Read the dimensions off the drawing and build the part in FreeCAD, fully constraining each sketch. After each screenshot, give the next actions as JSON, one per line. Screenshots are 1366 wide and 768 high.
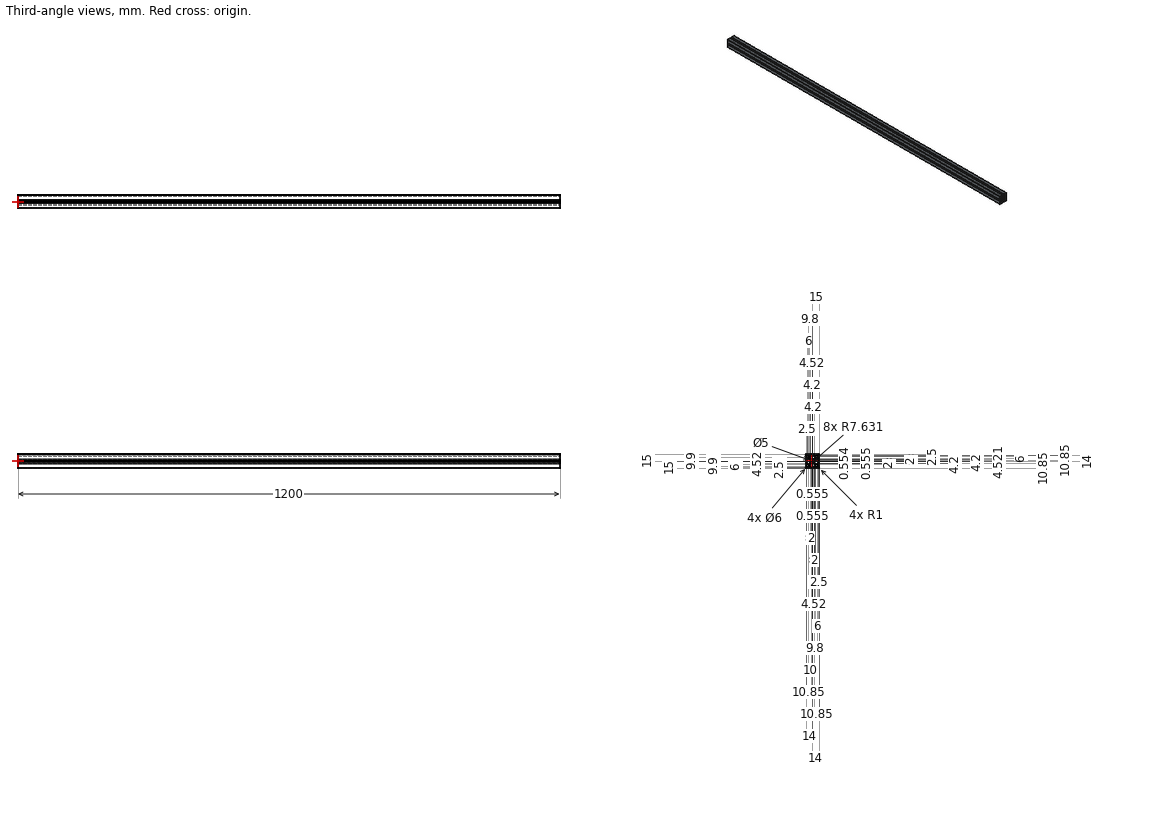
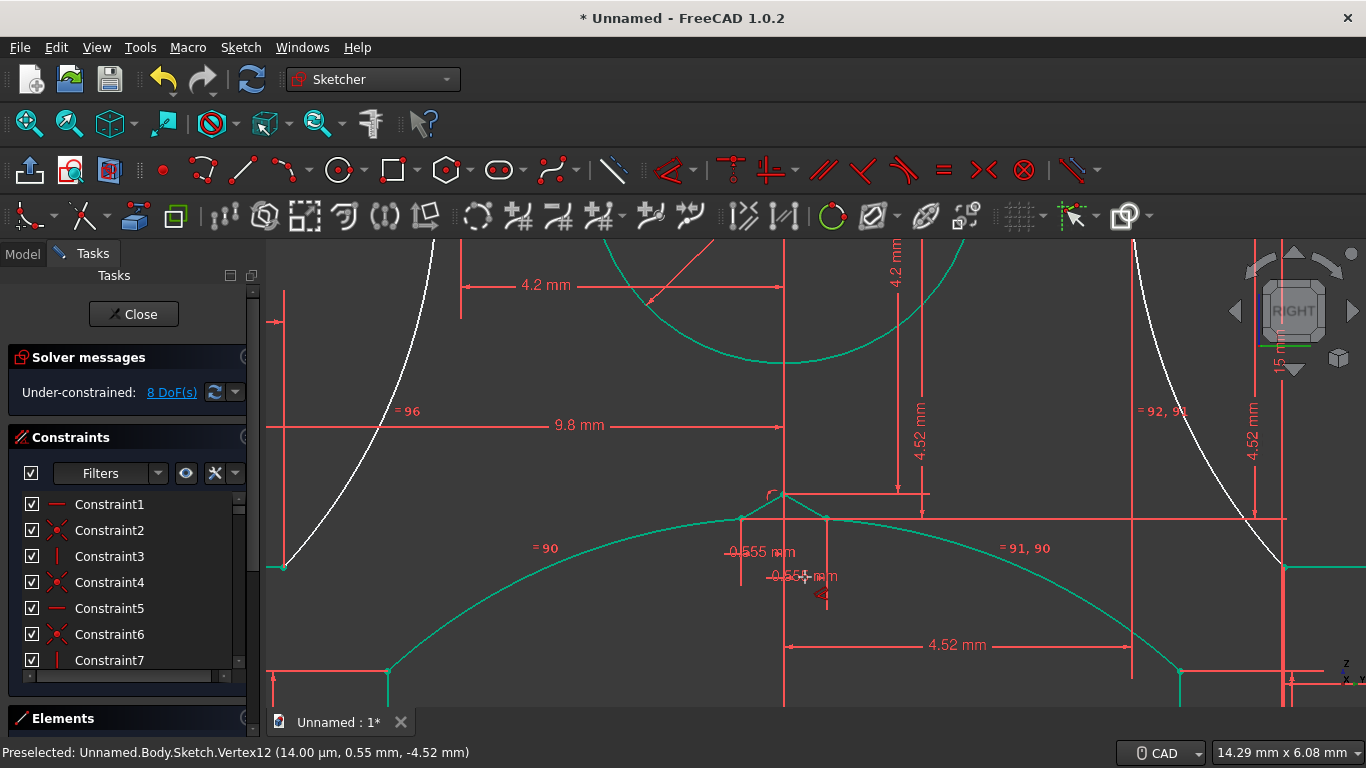
{"action": "scroll", "coordinate": [742, 520], "scroll_direction": "down", "scroll_amount": 10}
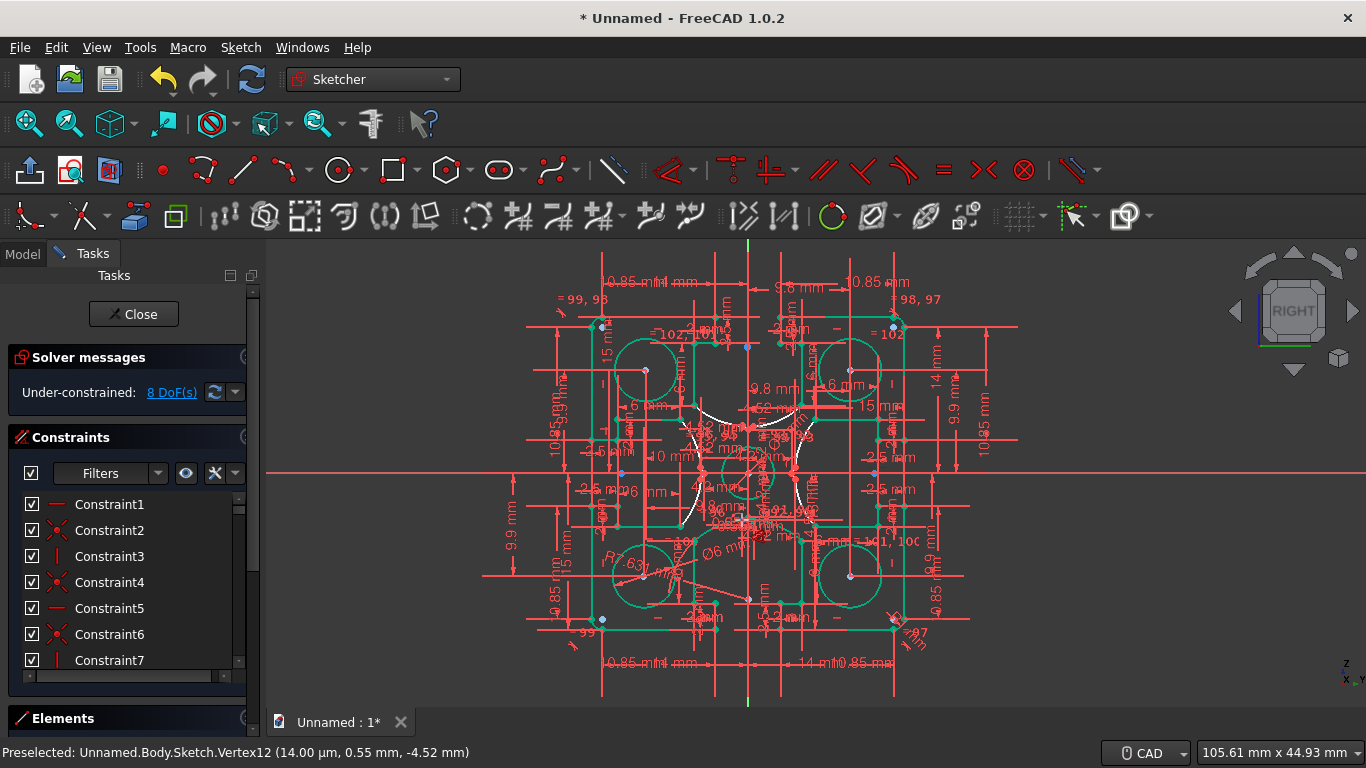
{"action": "scroll", "coordinate": [795, 479], "scroll_direction": "up", "scroll_amount": 10}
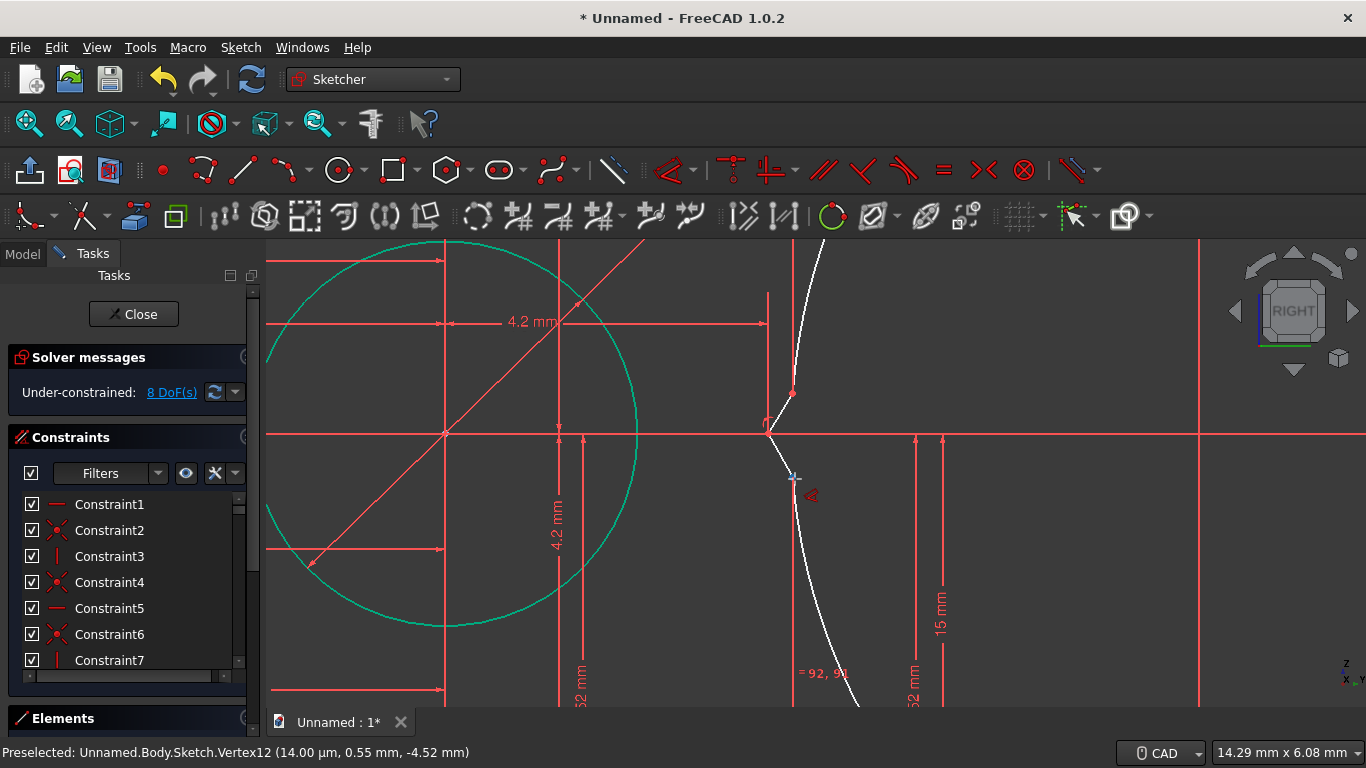
{"action": "left_click", "coordinate": [793, 477]}
{"action": "left_click", "coordinate": [827, 455]}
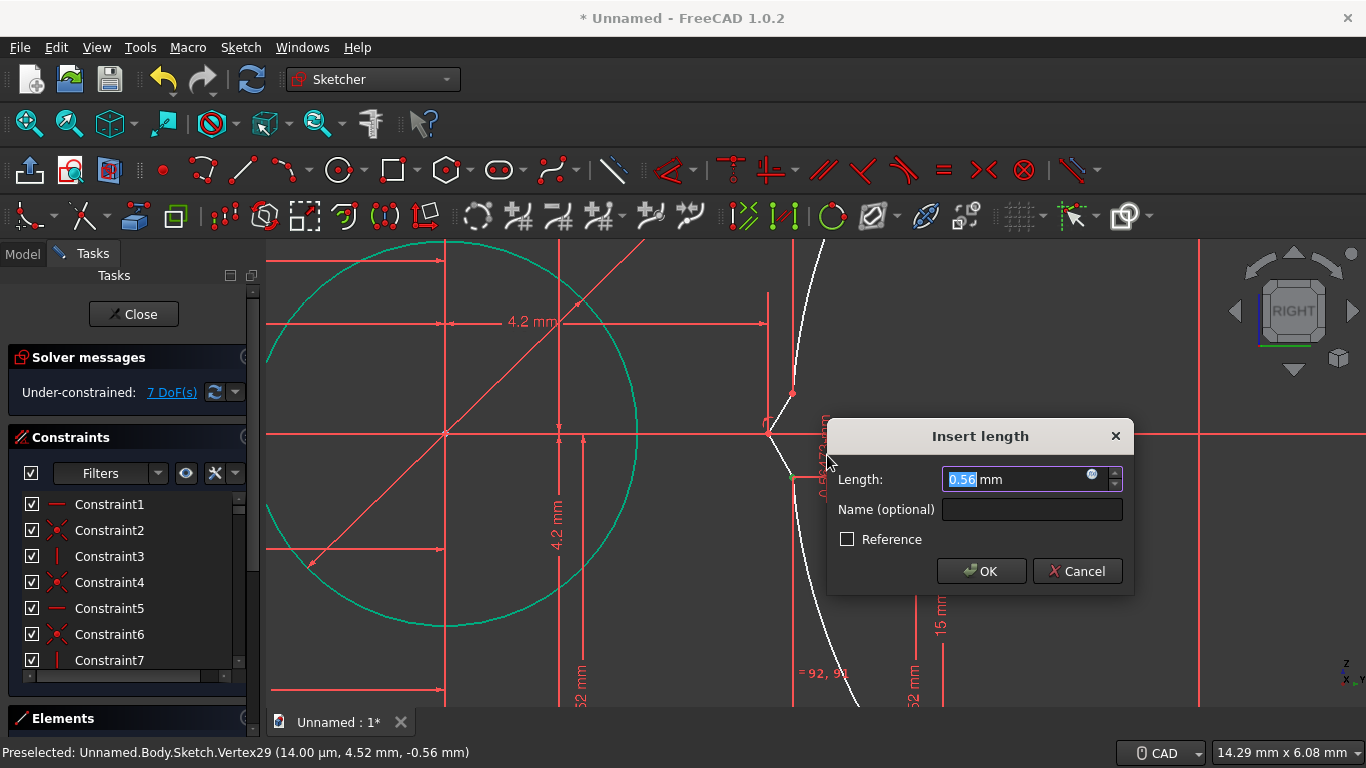
{"action": "type", "text": "0.554"}
{"action": "key", "text": "Return"}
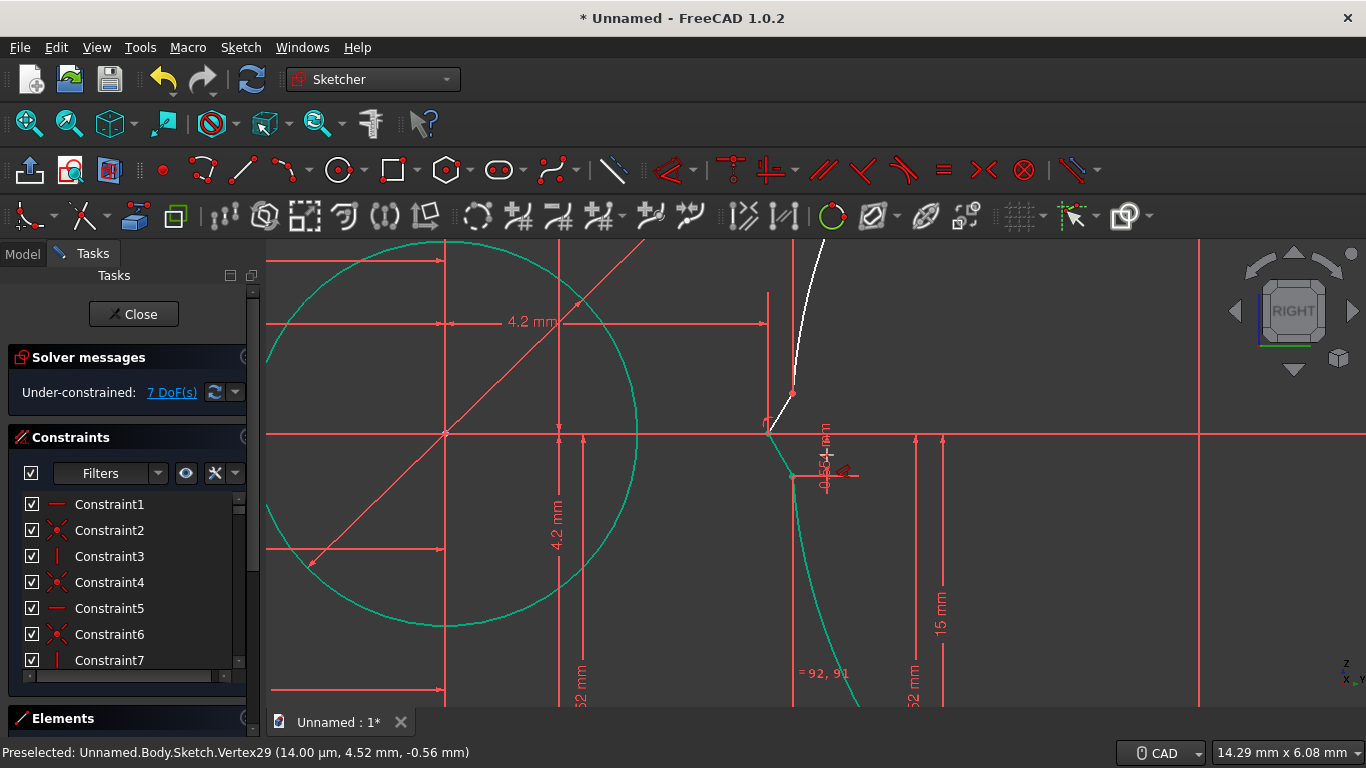
{"action": "left_click", "coordinate": [793, 393]}
{"action": "left_click", "coordinate": [827, 413]}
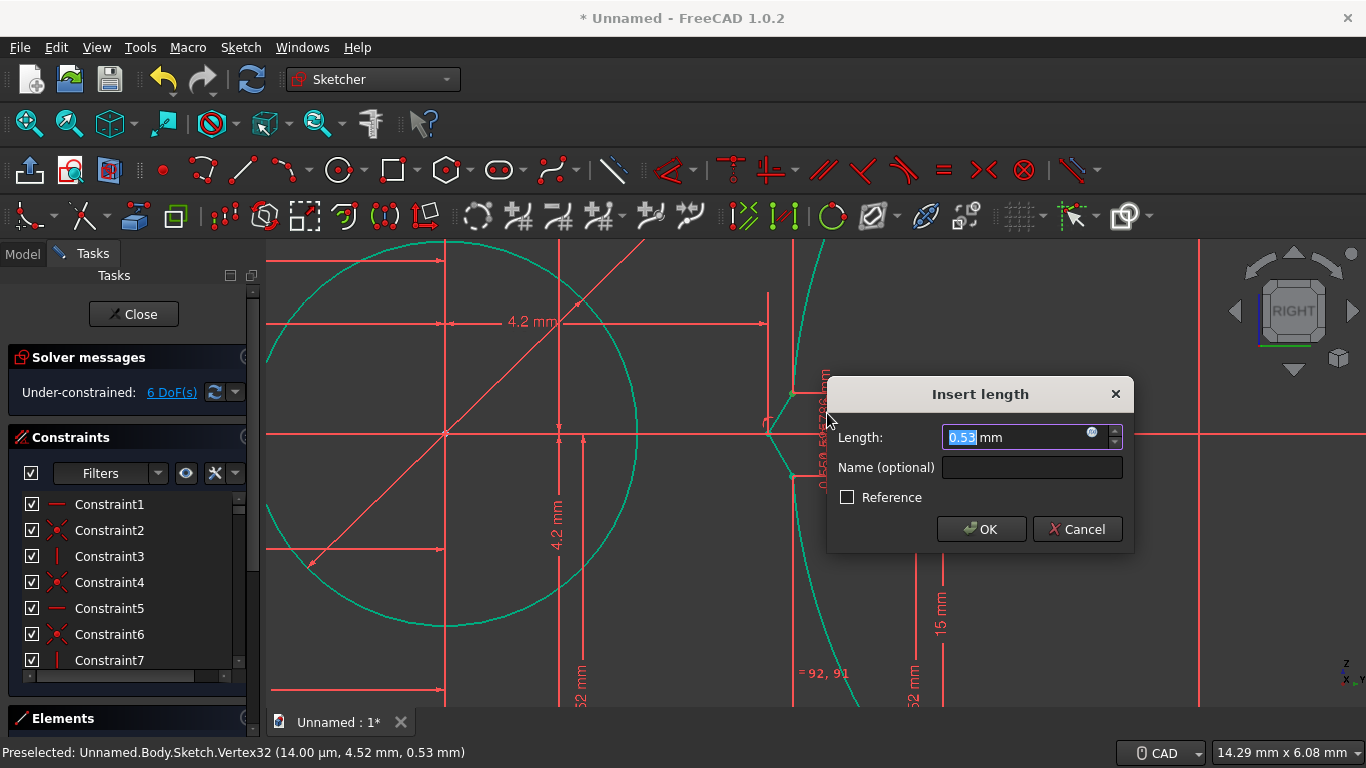
{"action": "type", "text": "0.555"}
{"action": "key", "text": "Return"}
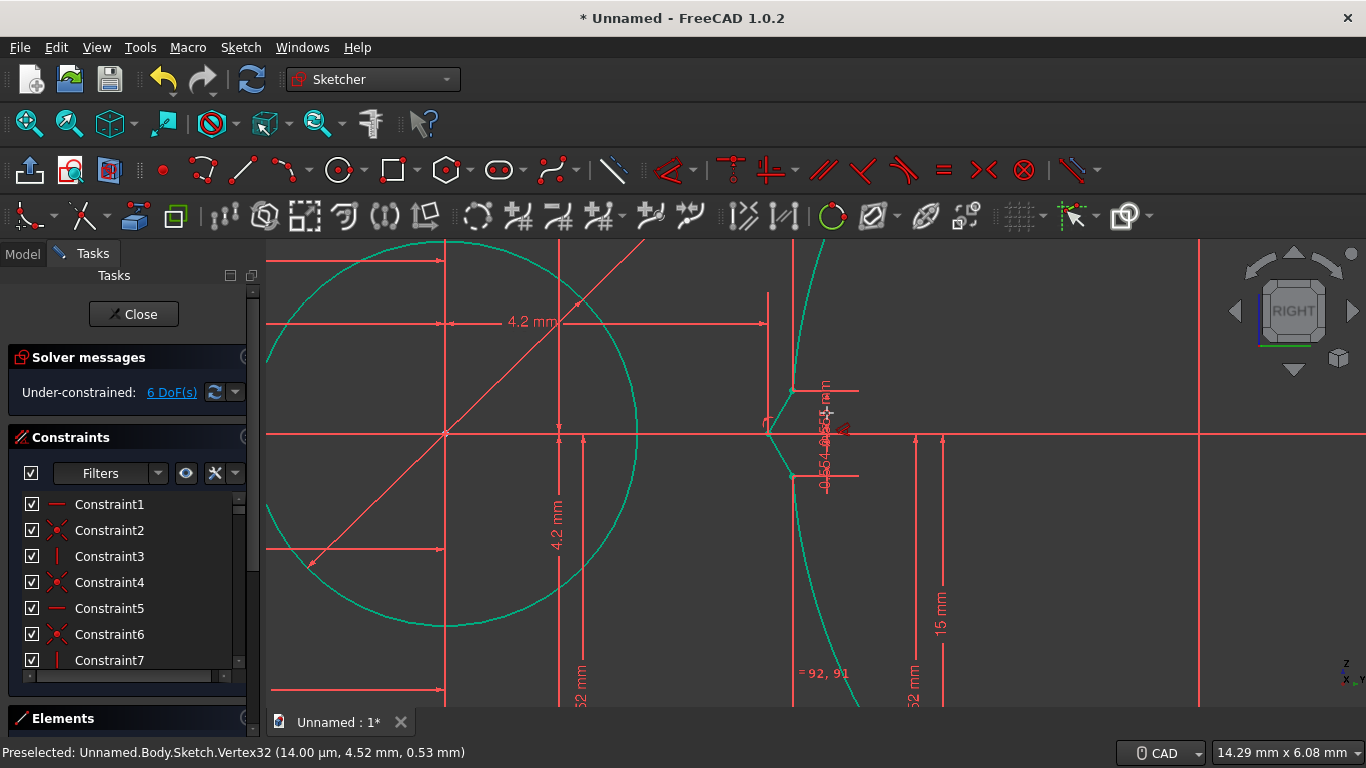
{"action": "scroll", "coordinate": [795, 479], "scroll_direction": "down", "scroll_amount": 10}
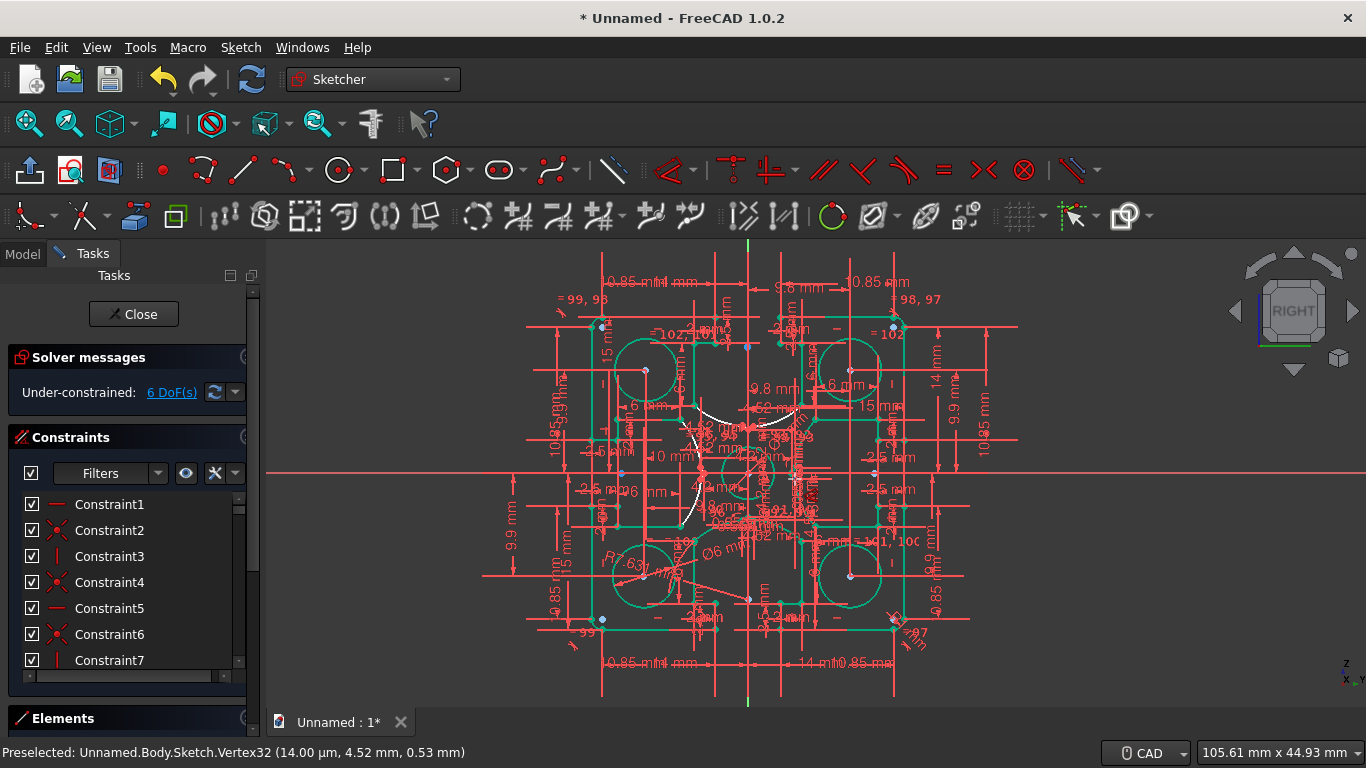
{"action": "scroll", "coordinate": [754, 427], "scroll_direction": "up", "scroll_amount": 10}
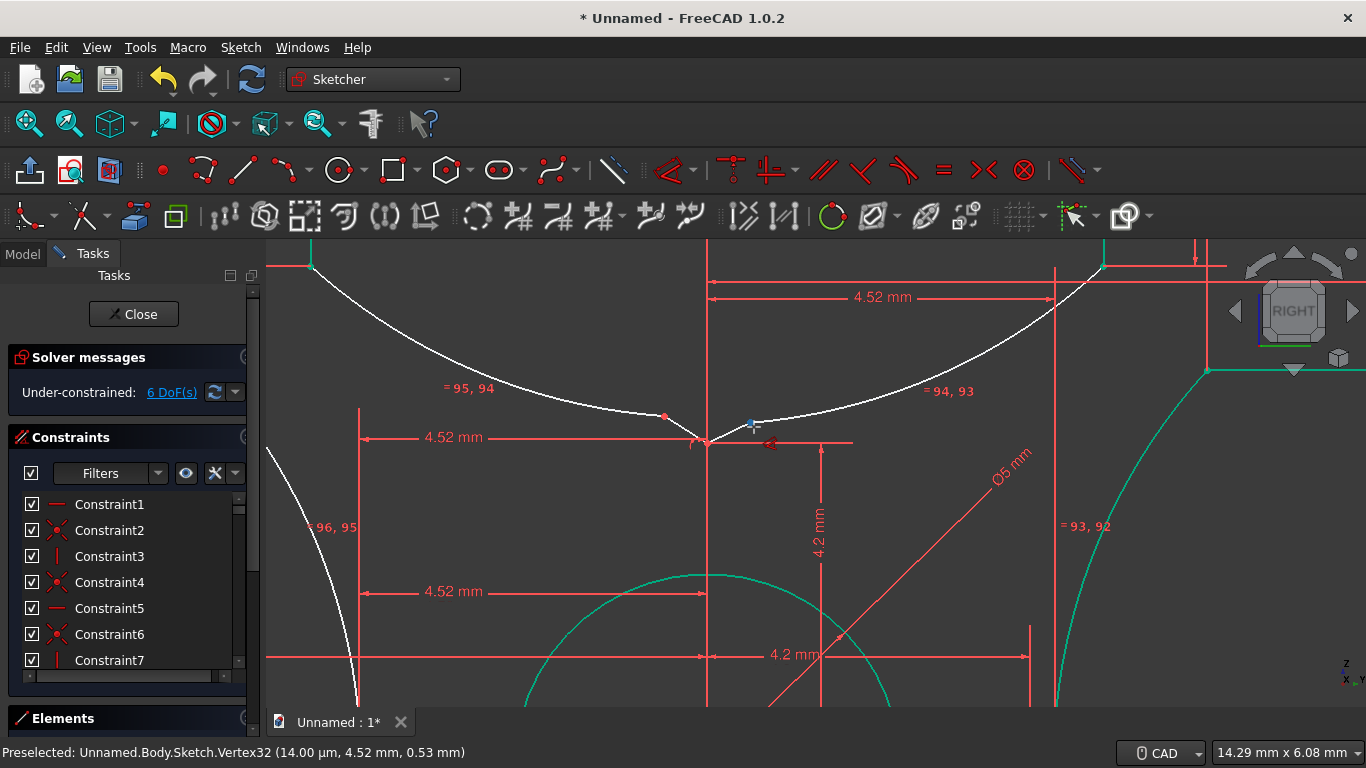
{"action": "left_click", "coordinate": [750, 423]}
{"action": "left_click", "coordinate": [729, 389]}